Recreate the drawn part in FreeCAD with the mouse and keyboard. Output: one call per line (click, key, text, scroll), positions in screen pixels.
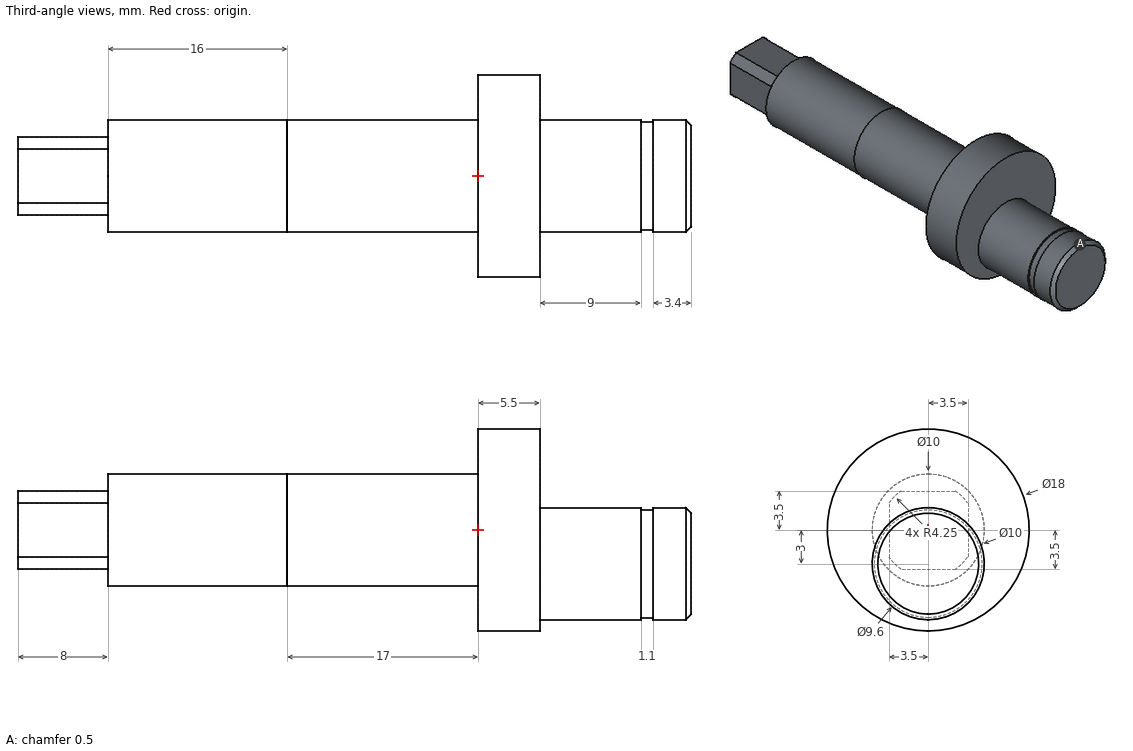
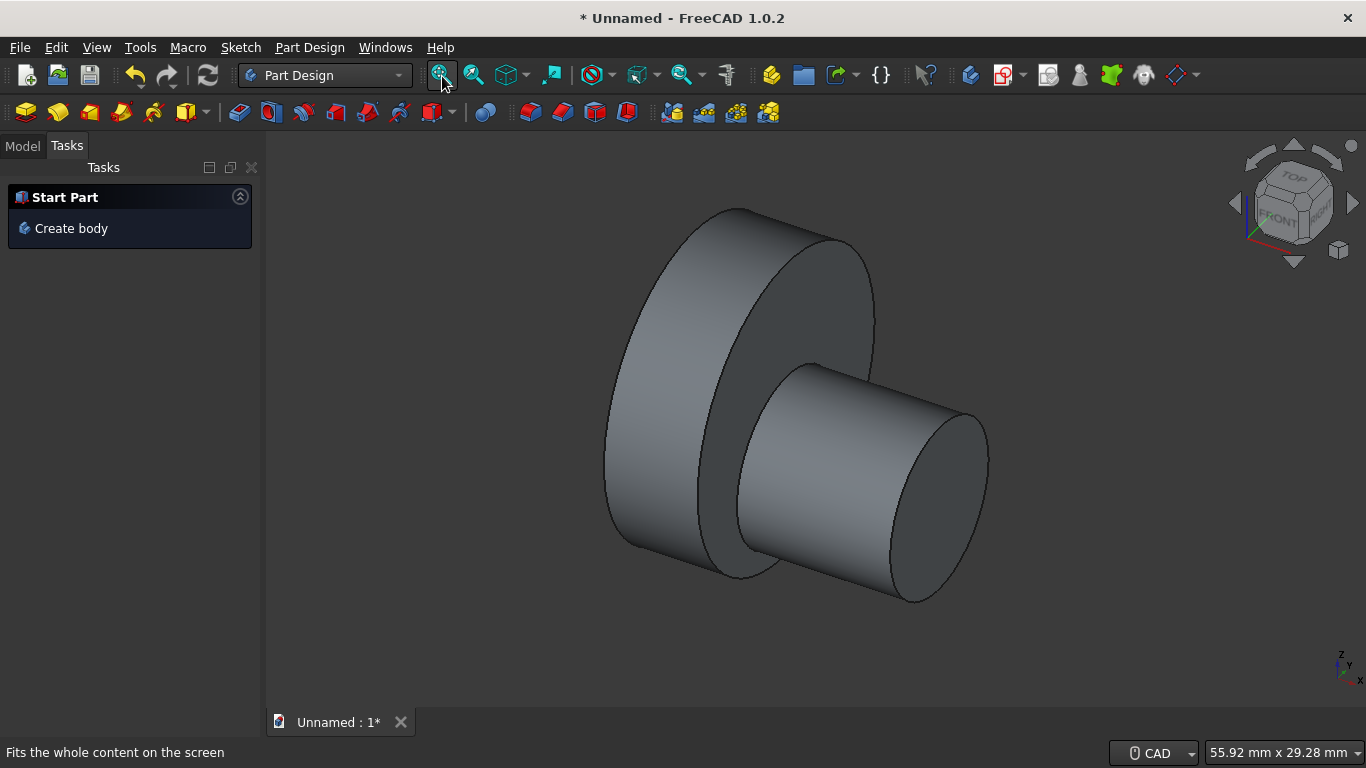
click(939, 507)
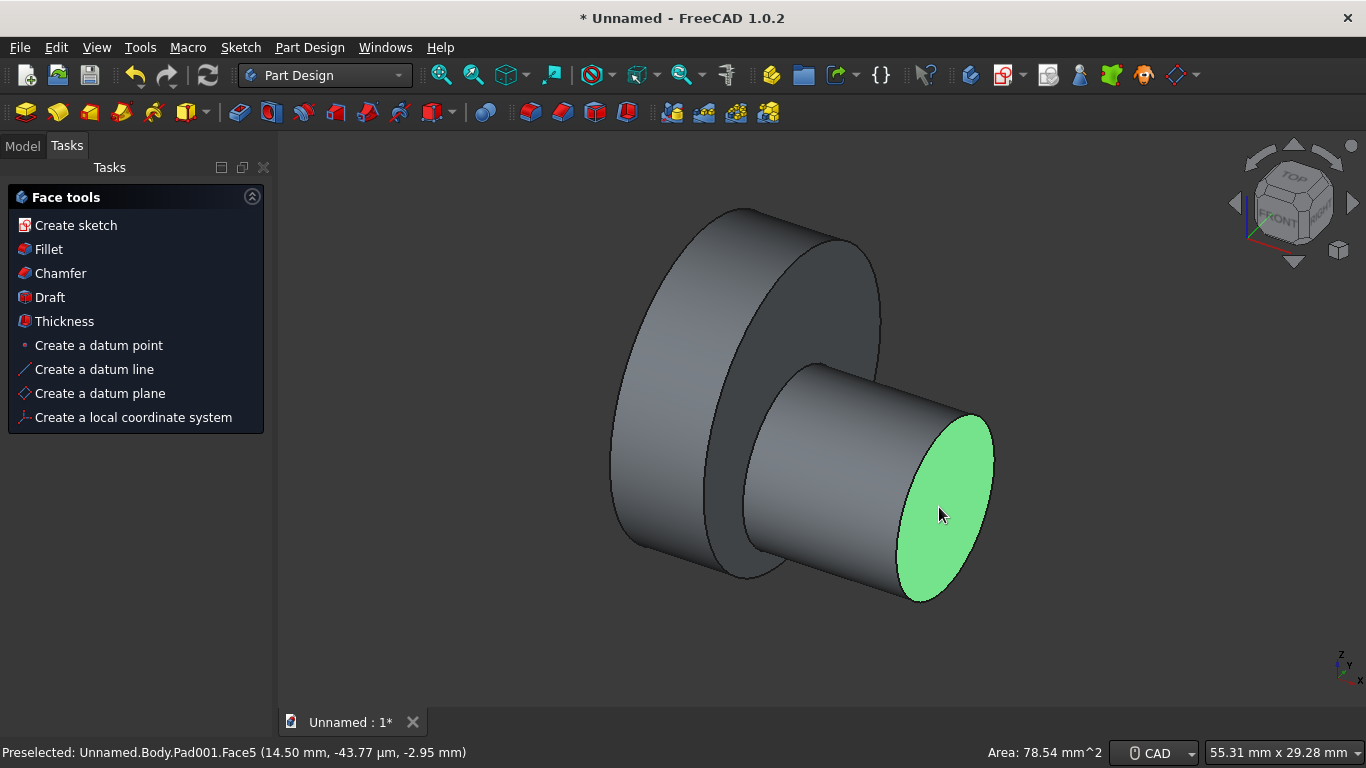
click(1004, 76)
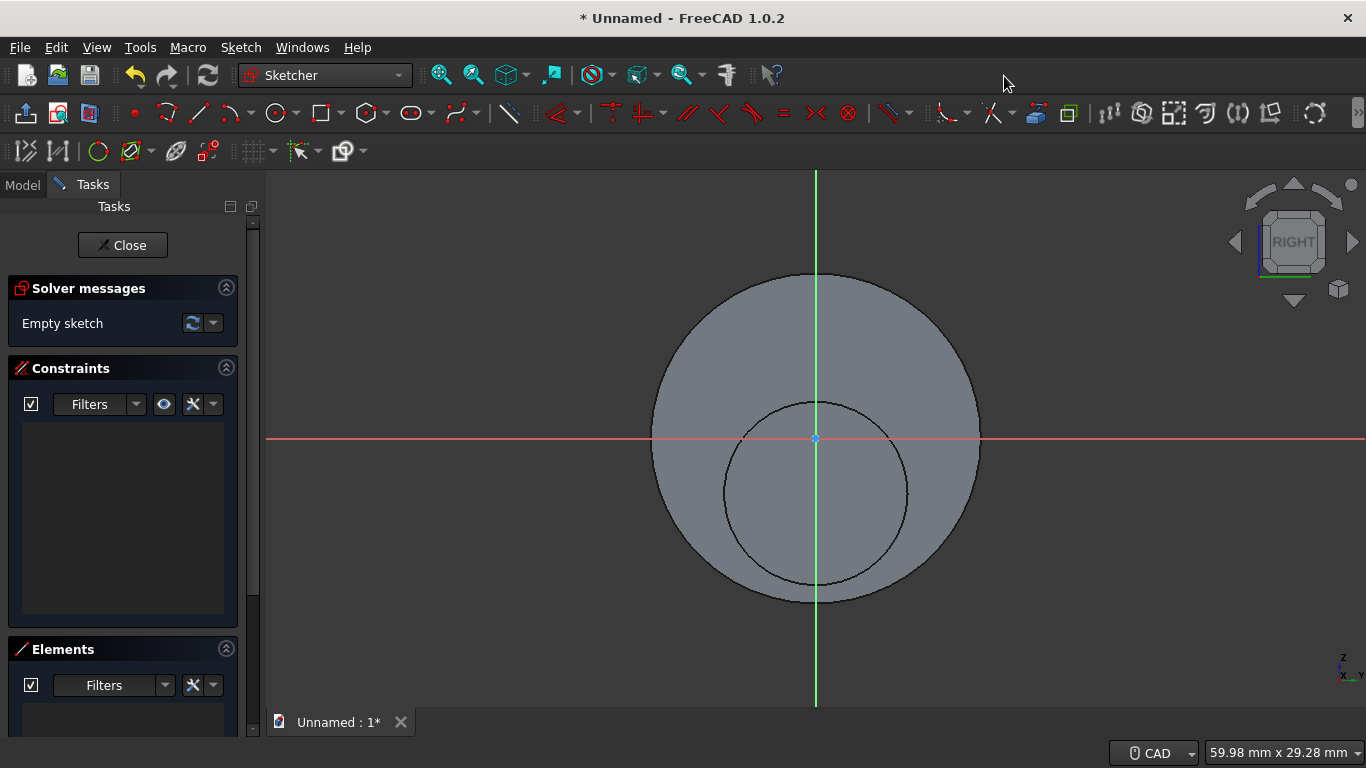
scroll(899, 560, up, 3)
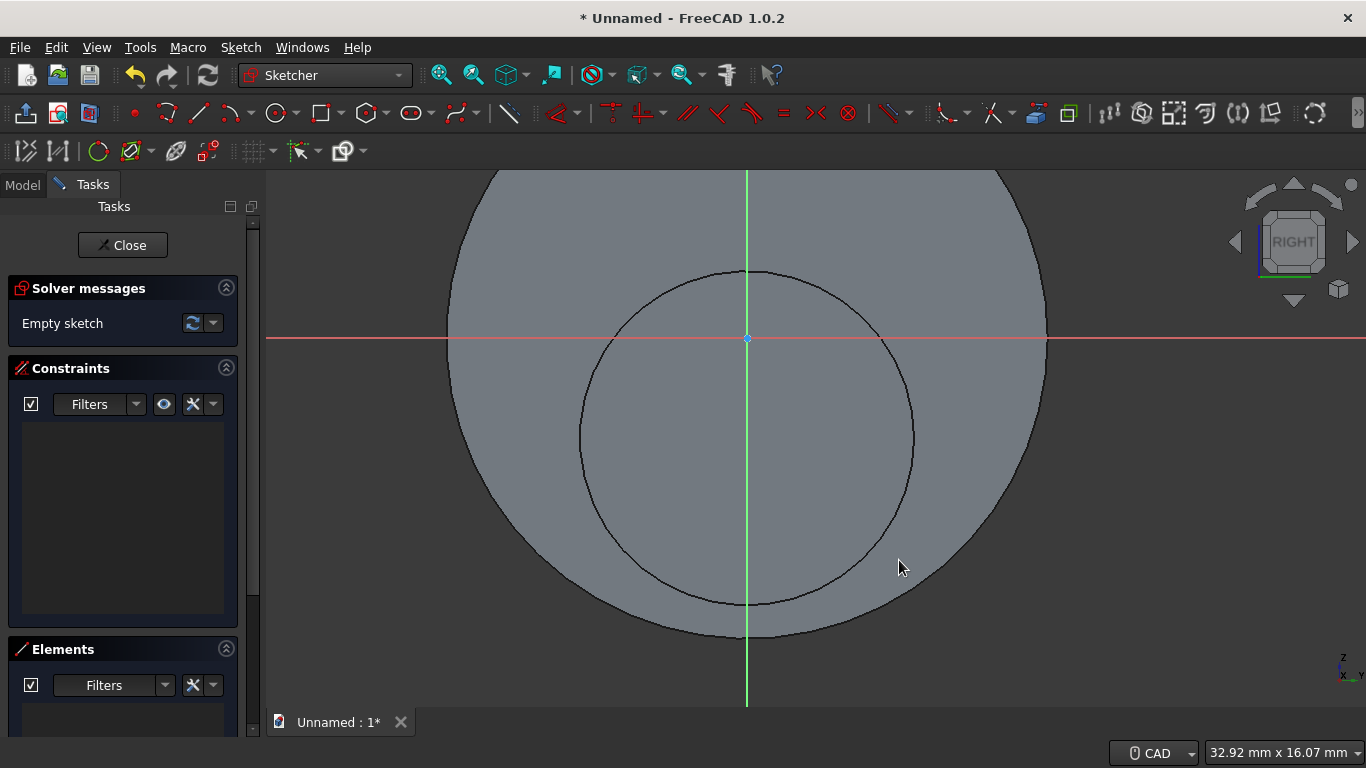
click(276, 114)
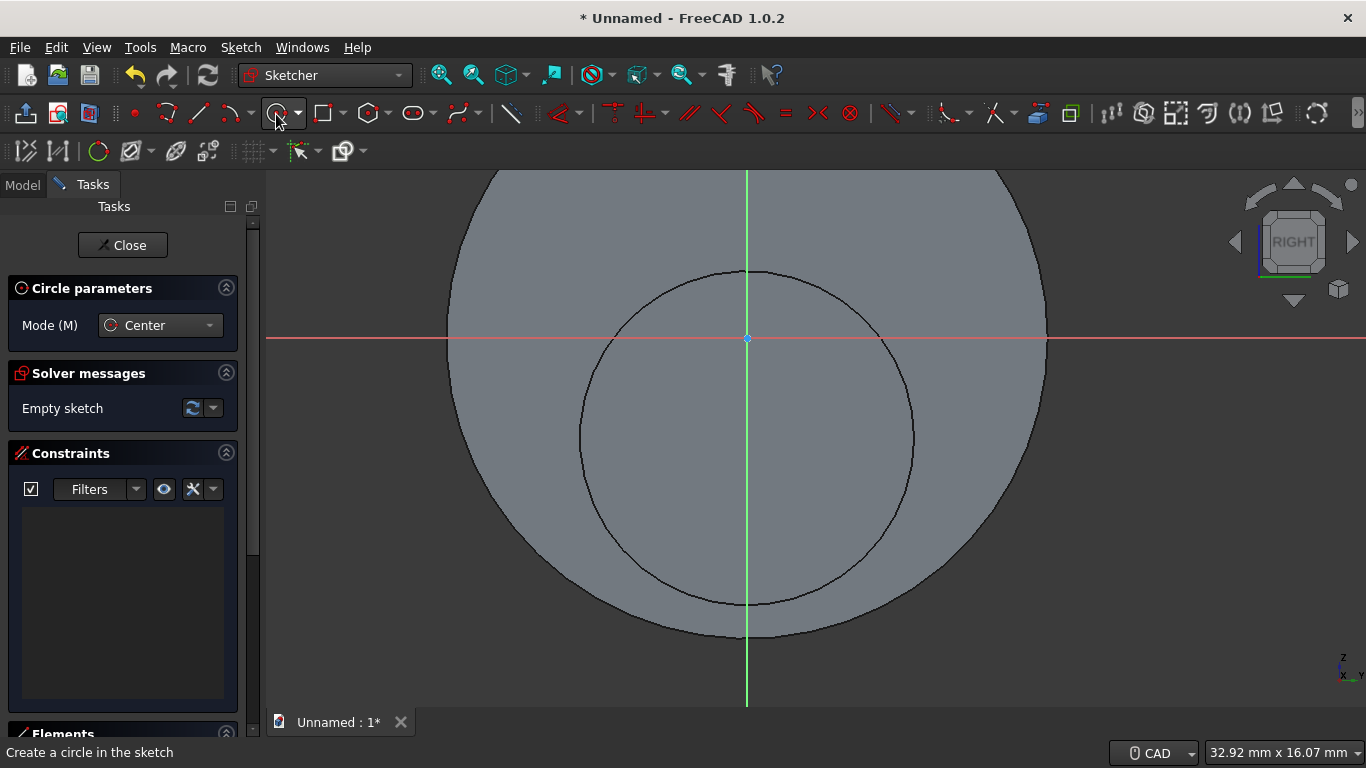
click(747, 438)
click(860, 552)
key(Escape)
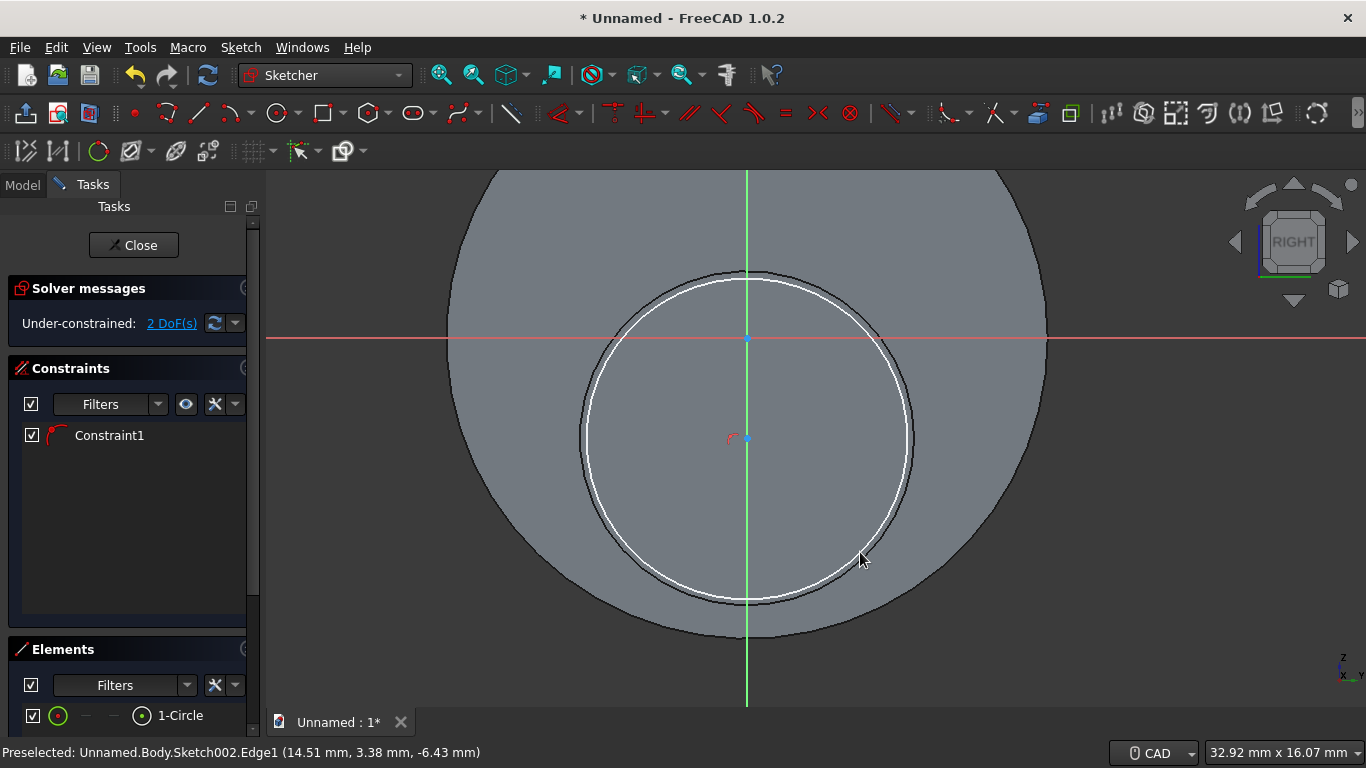
key(d)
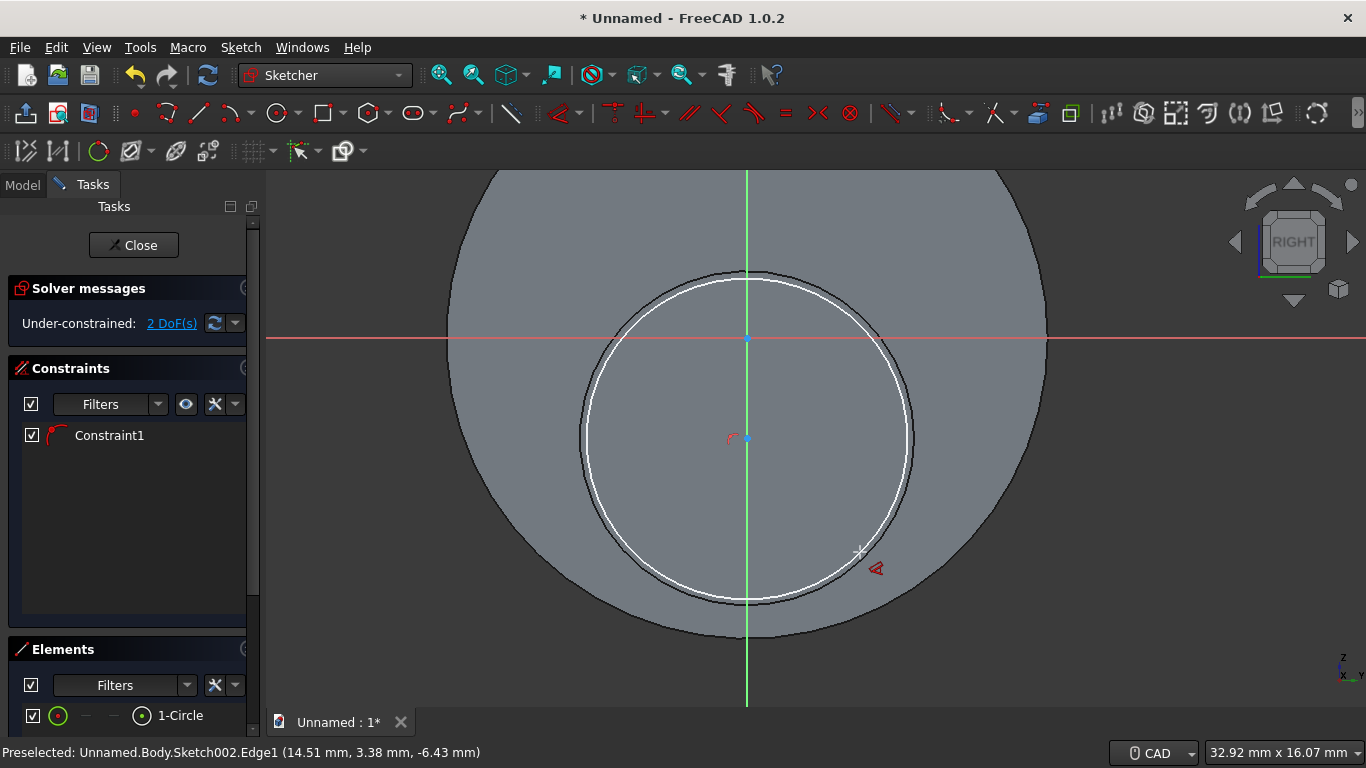
click(860, 325)
click(883, 302)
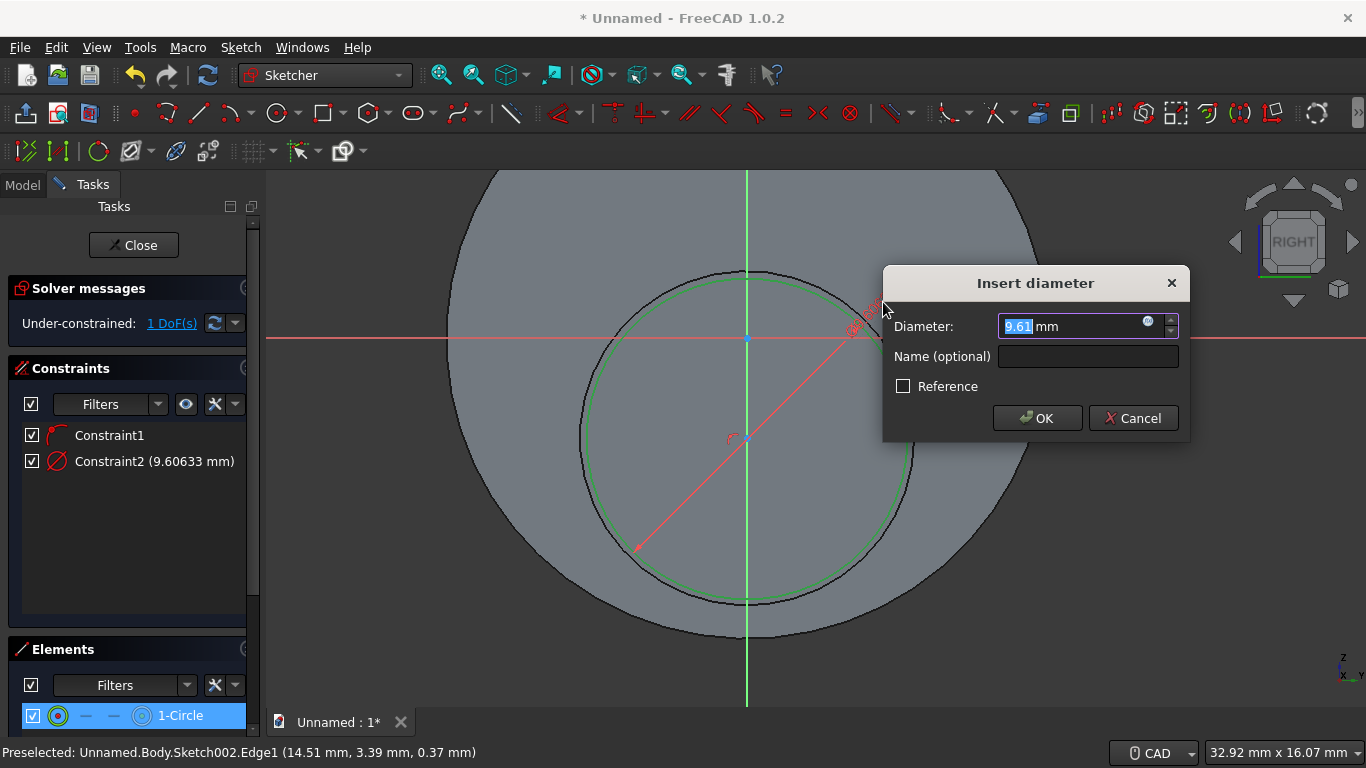
text(9.6)
key(Return)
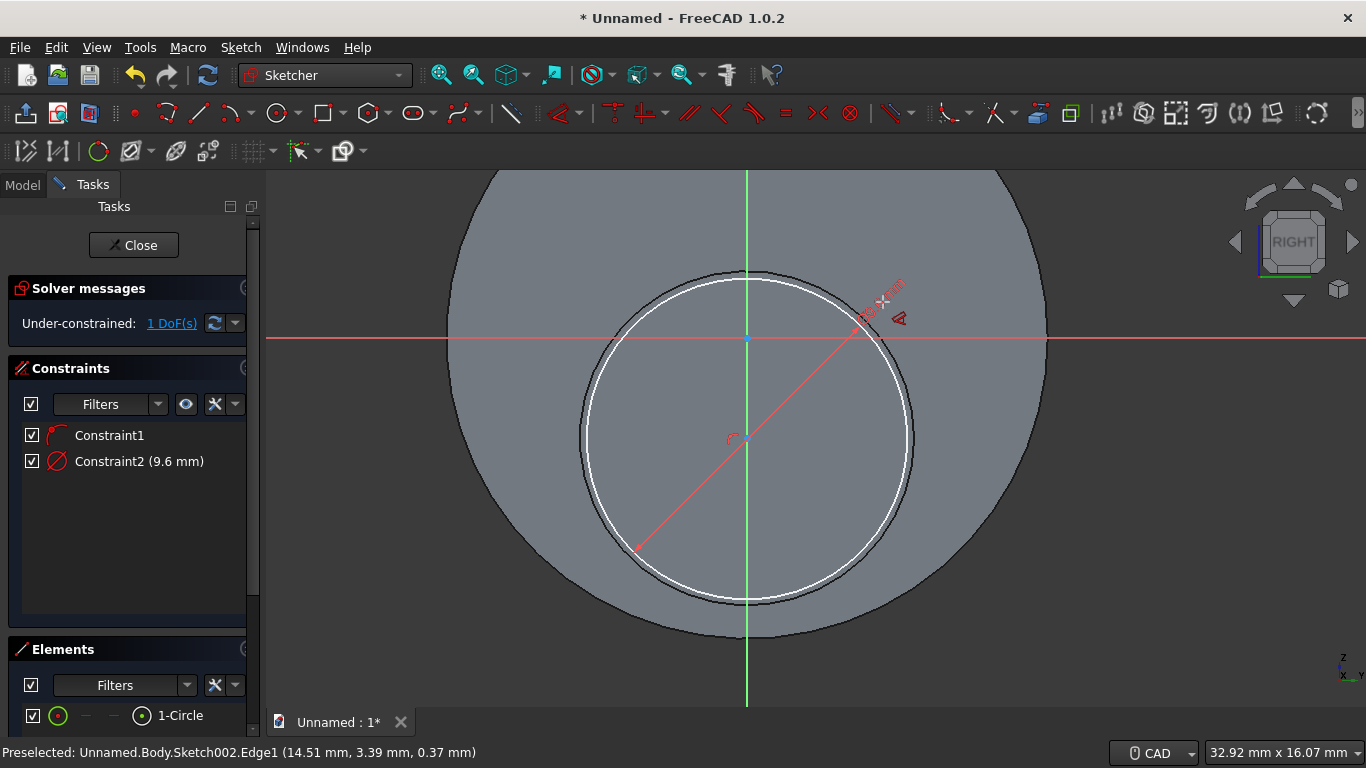
click(747, 439)
click(781, 389)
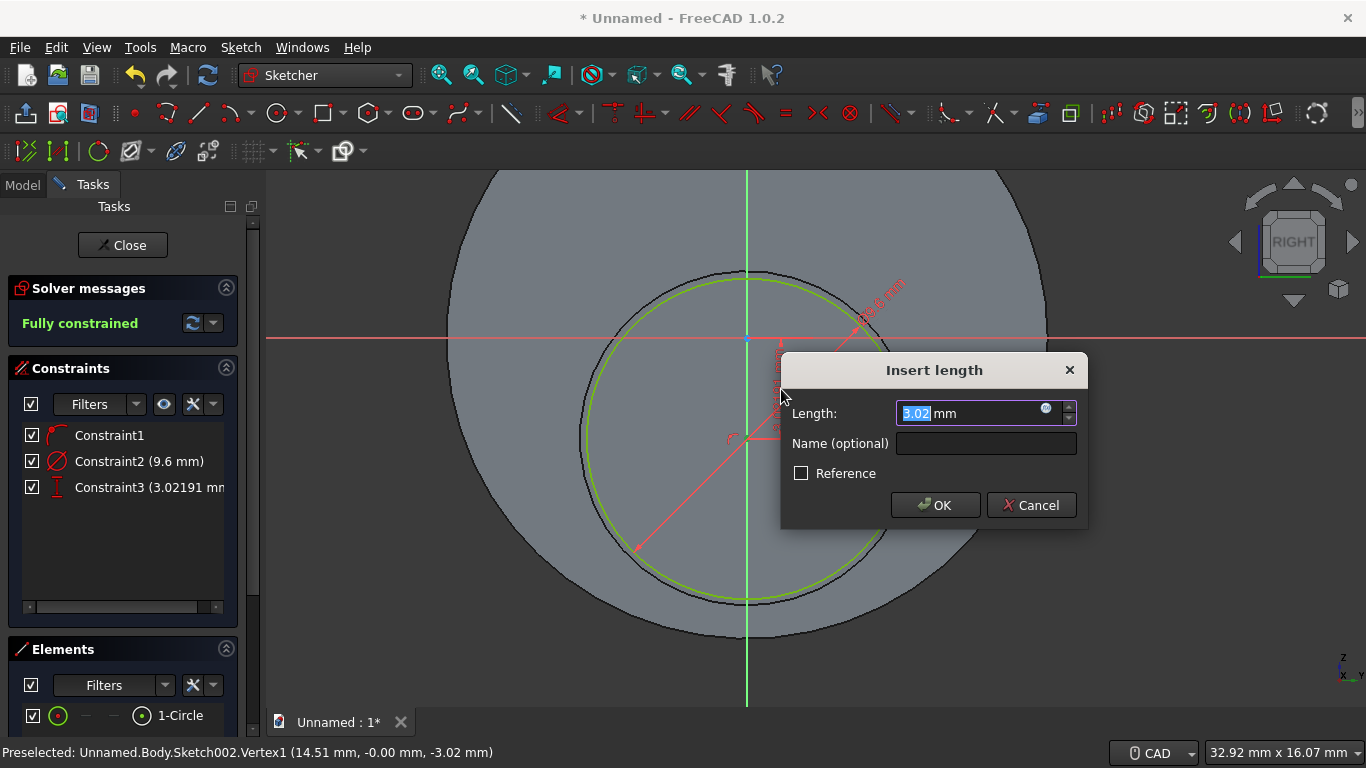
text(3)
key(Return)
key(Escape)